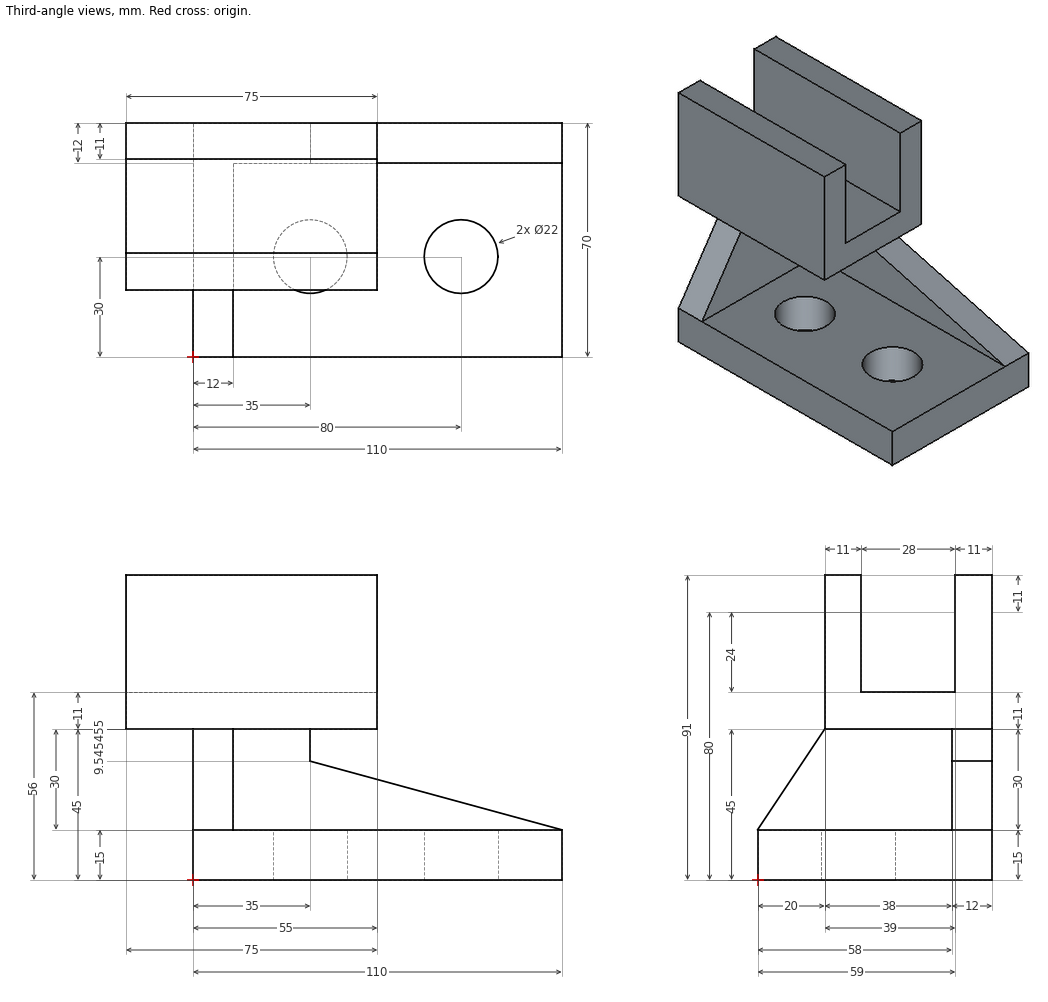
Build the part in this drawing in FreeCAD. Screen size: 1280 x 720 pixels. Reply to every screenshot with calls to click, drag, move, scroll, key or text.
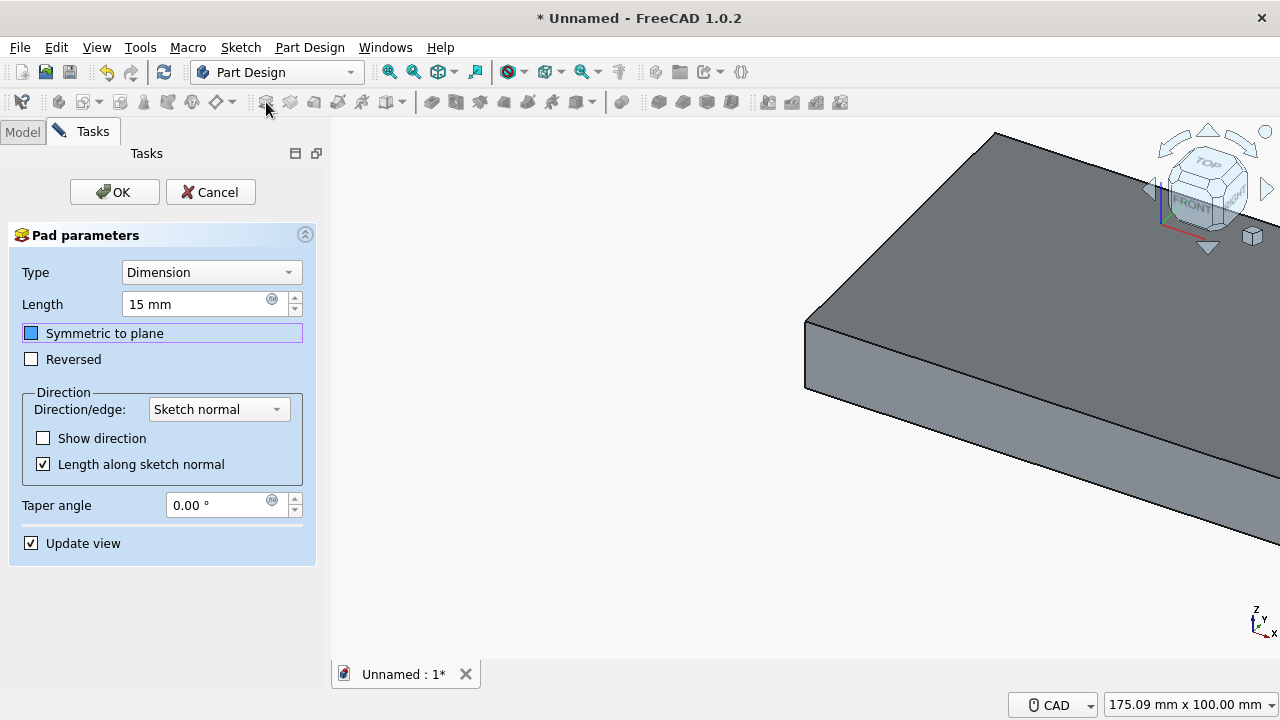
click(115, 192)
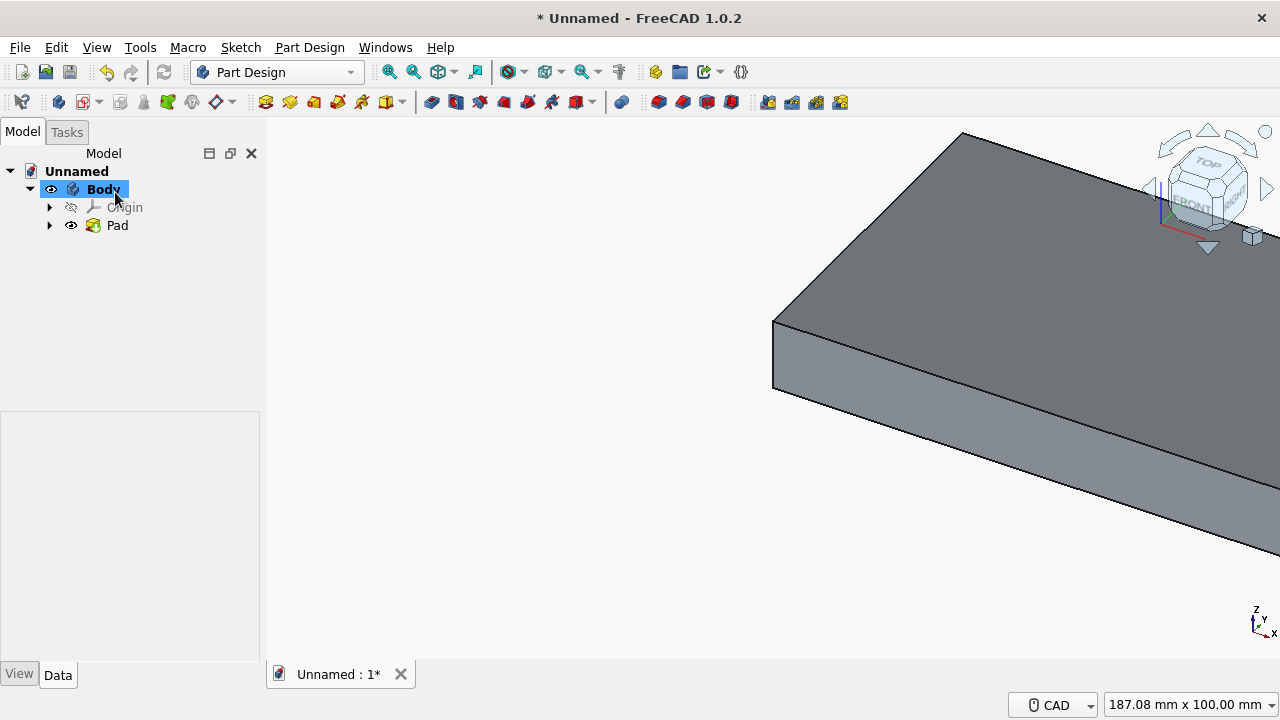
click(390, 72)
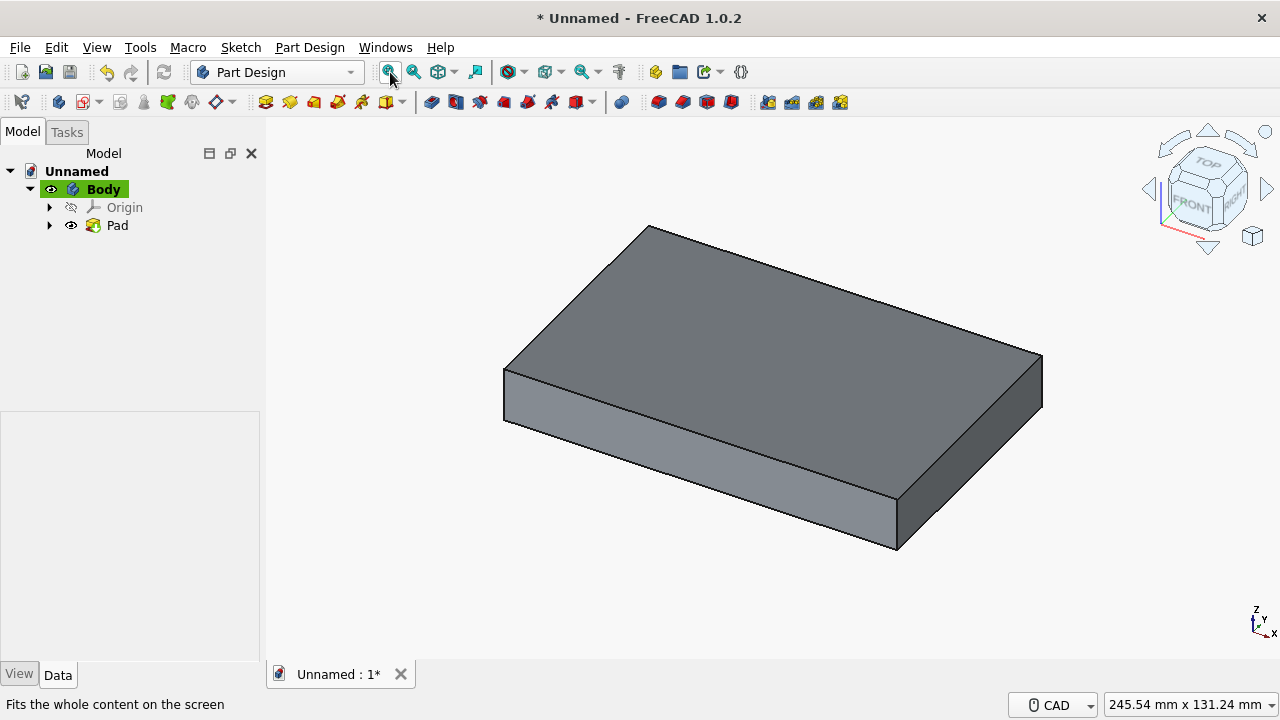
key(4)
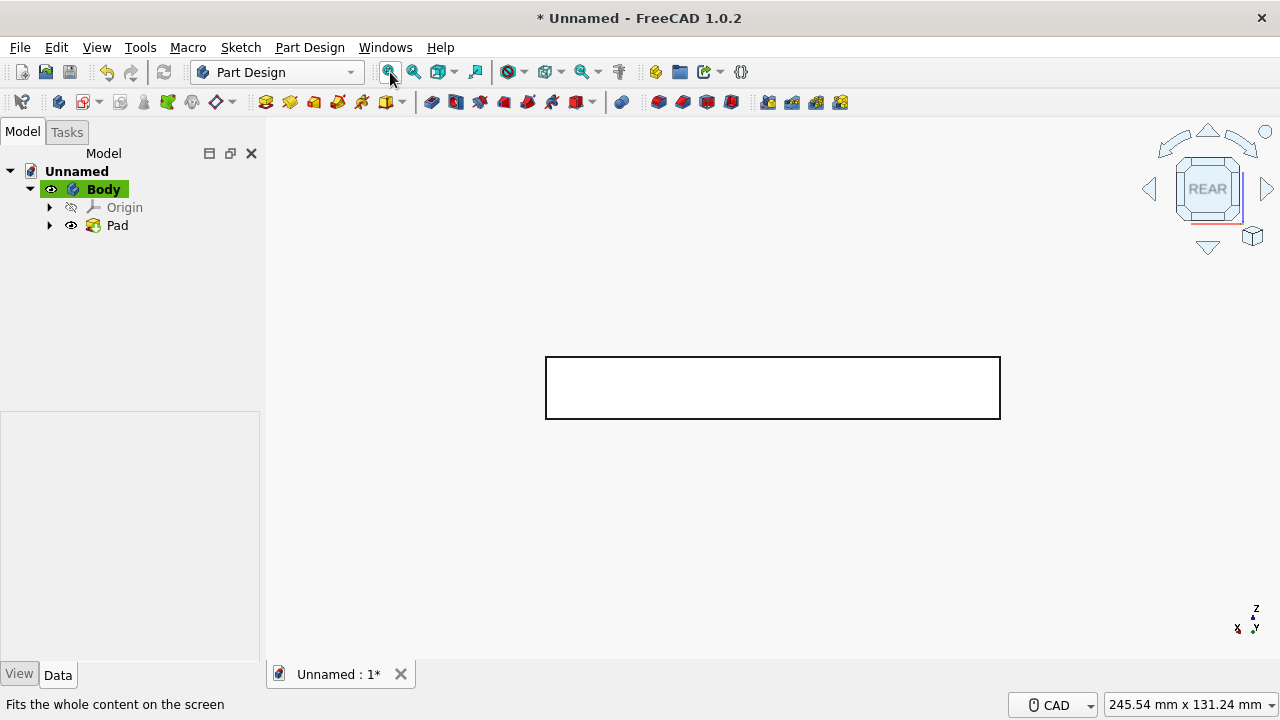
click(390, 72)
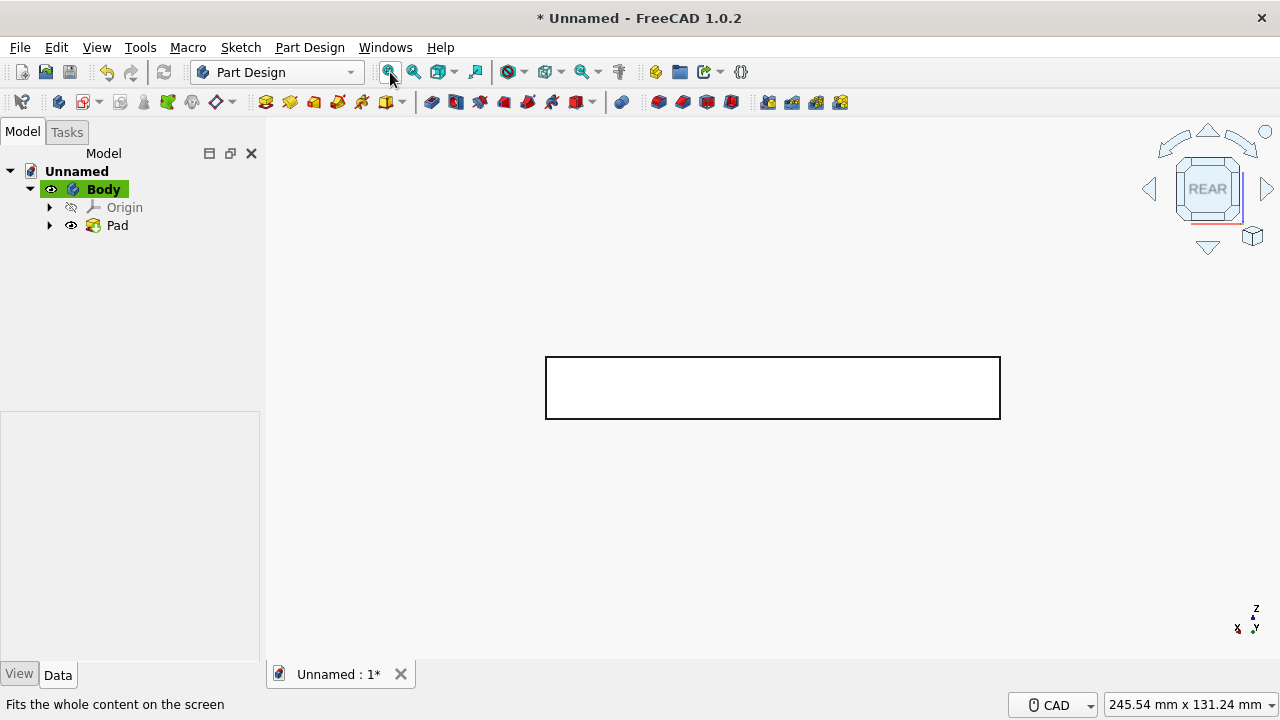
click(578, 387)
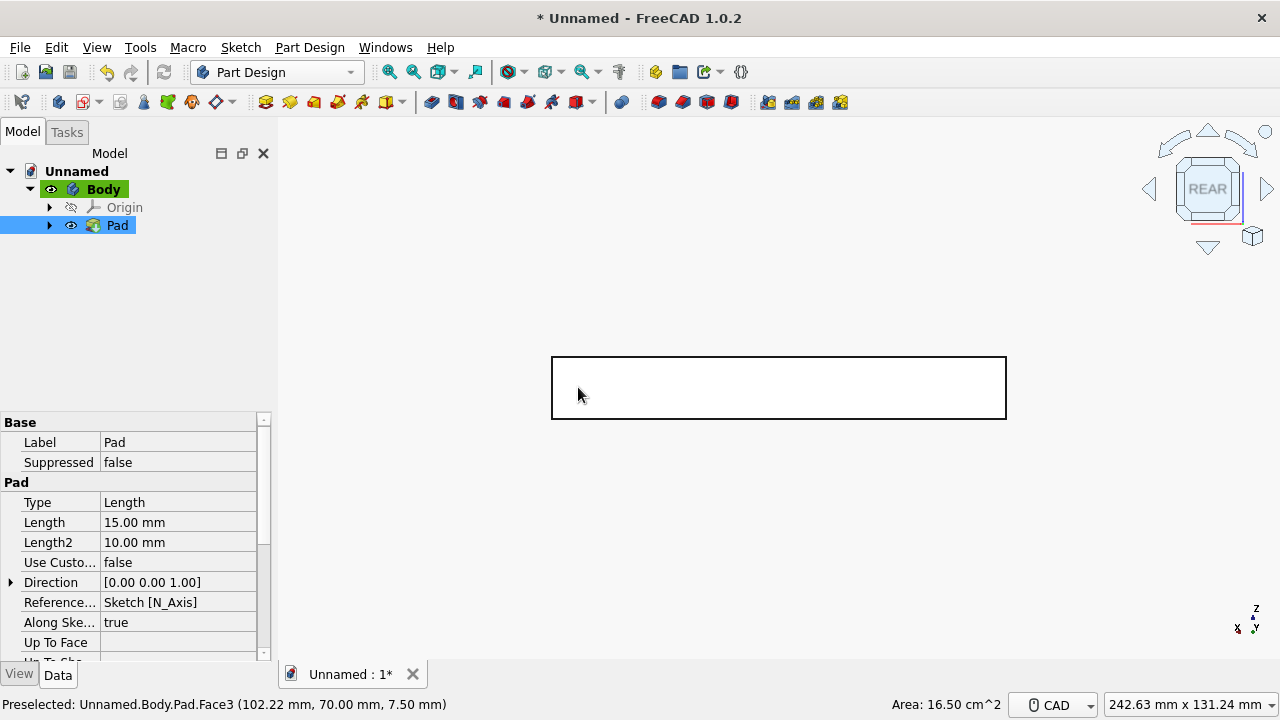
click(84, 102)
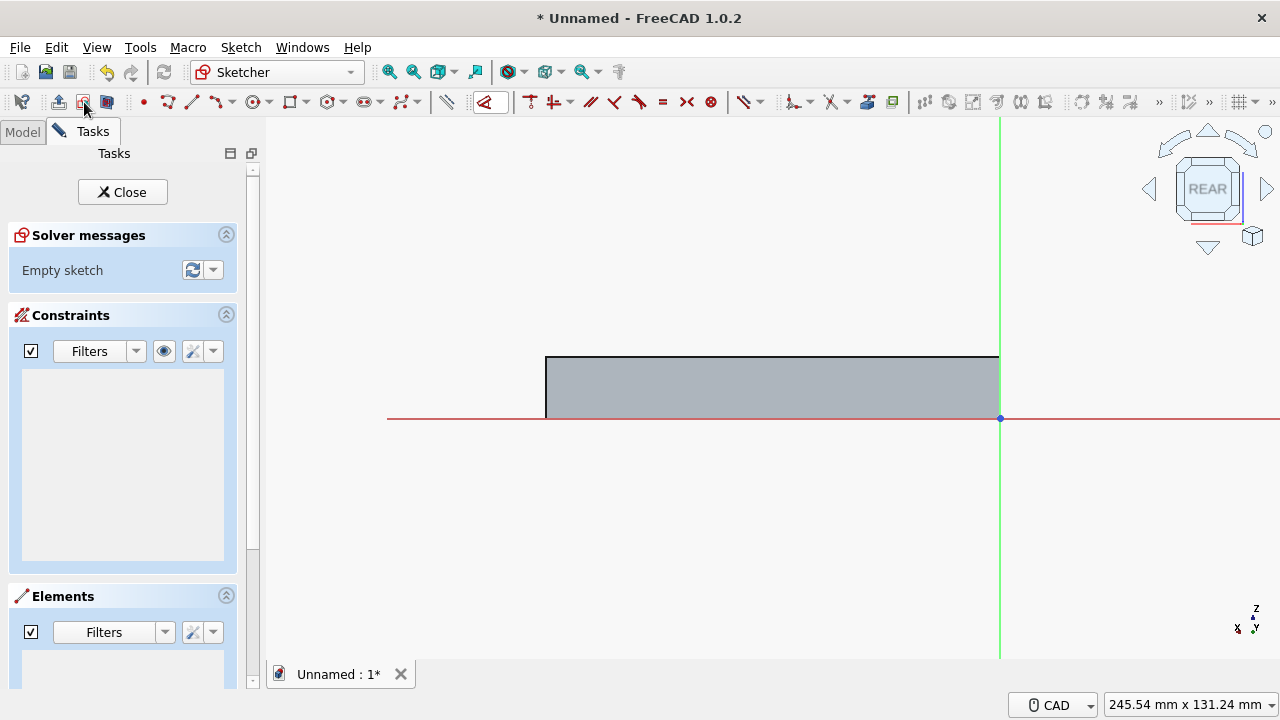
key(g)
key(m)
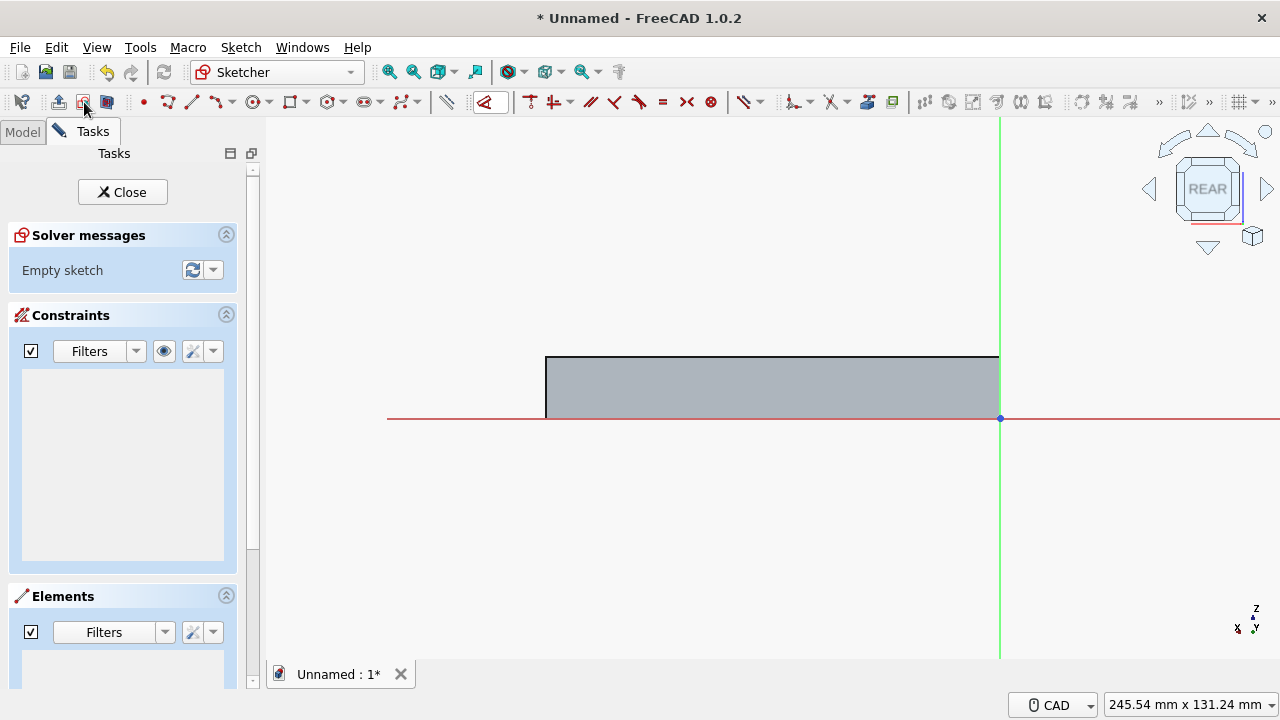
click(1000, 357)
click(991, 233)
click(546, 357)
click(1000, 358)
key(Escape)
key(Escape)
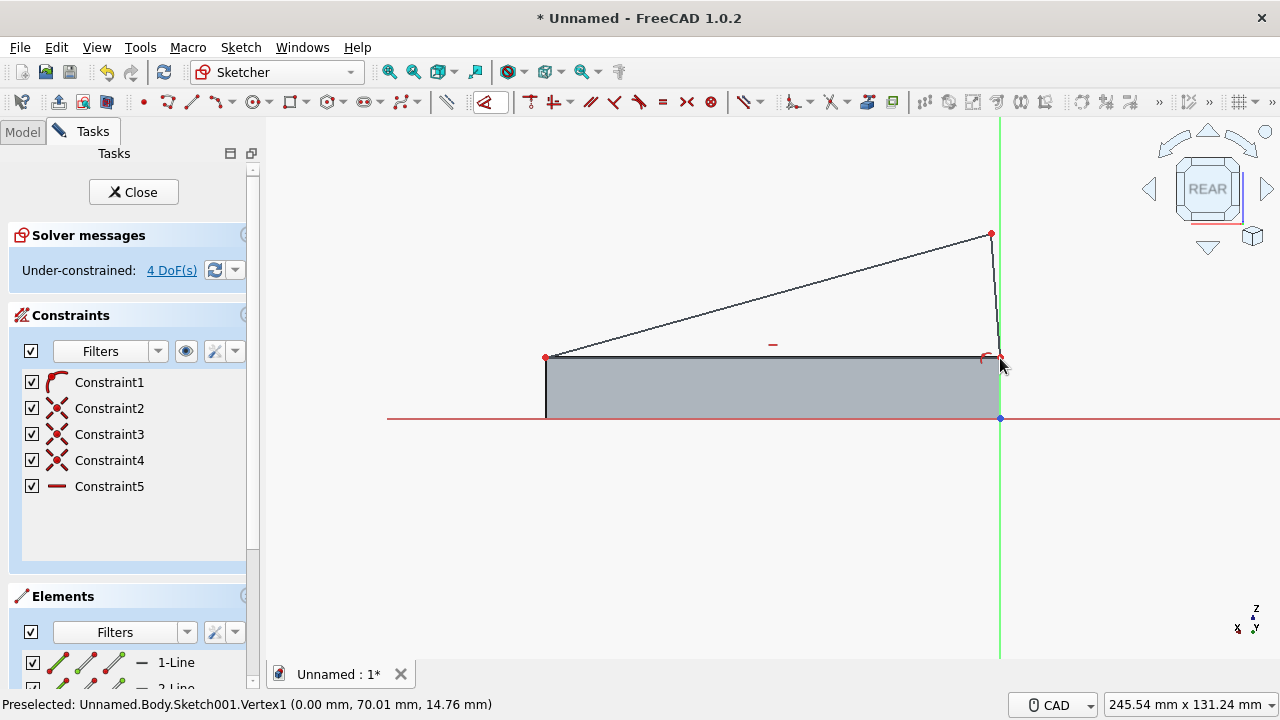
click(997, 321)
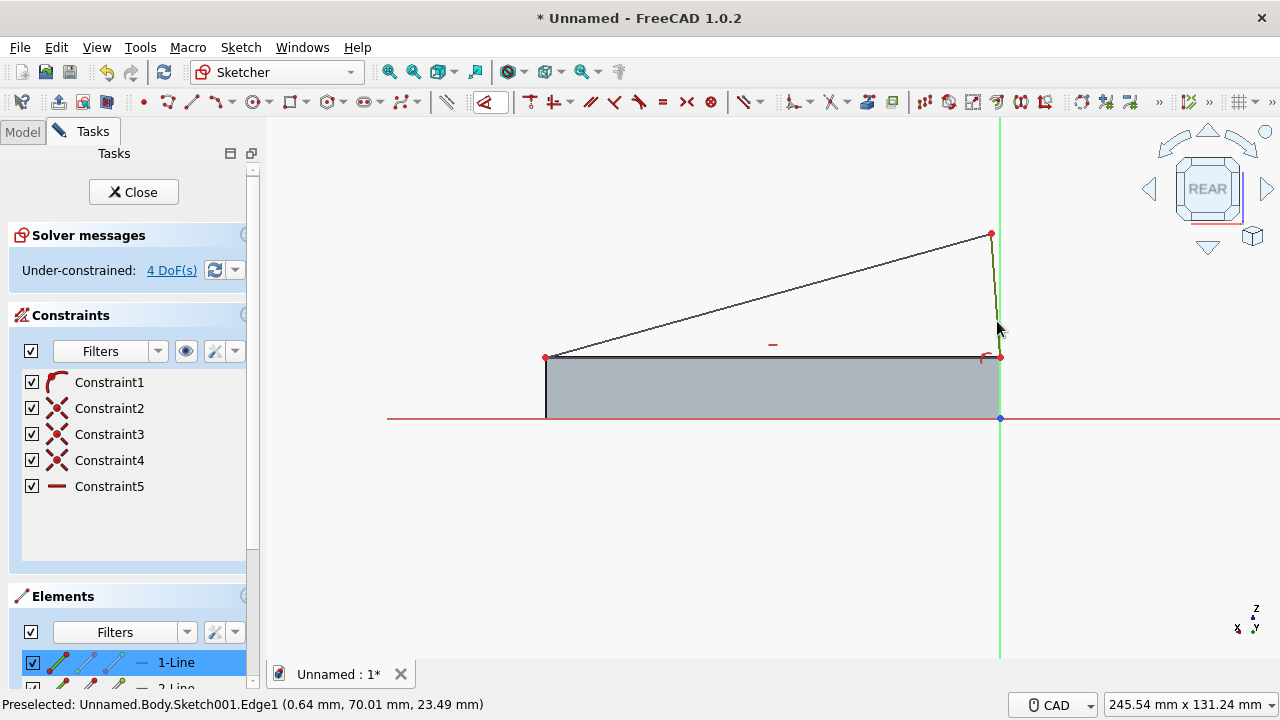
key(v)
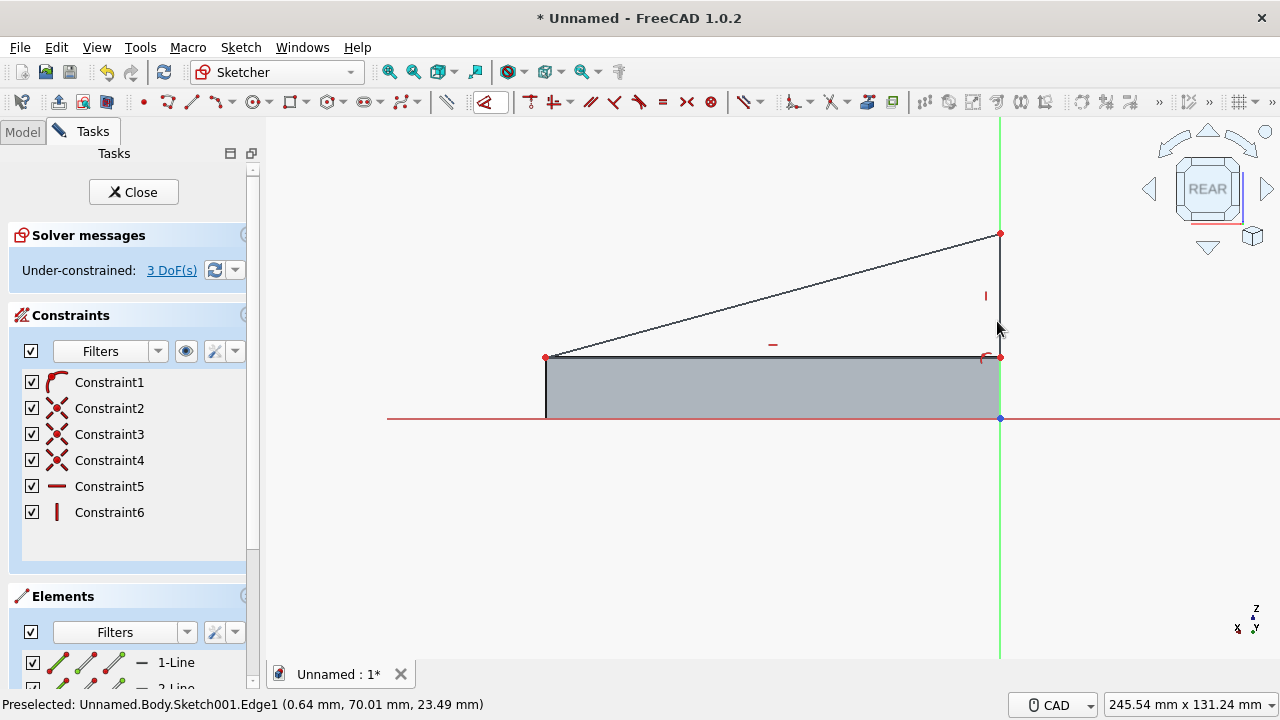
click(1000, 321)